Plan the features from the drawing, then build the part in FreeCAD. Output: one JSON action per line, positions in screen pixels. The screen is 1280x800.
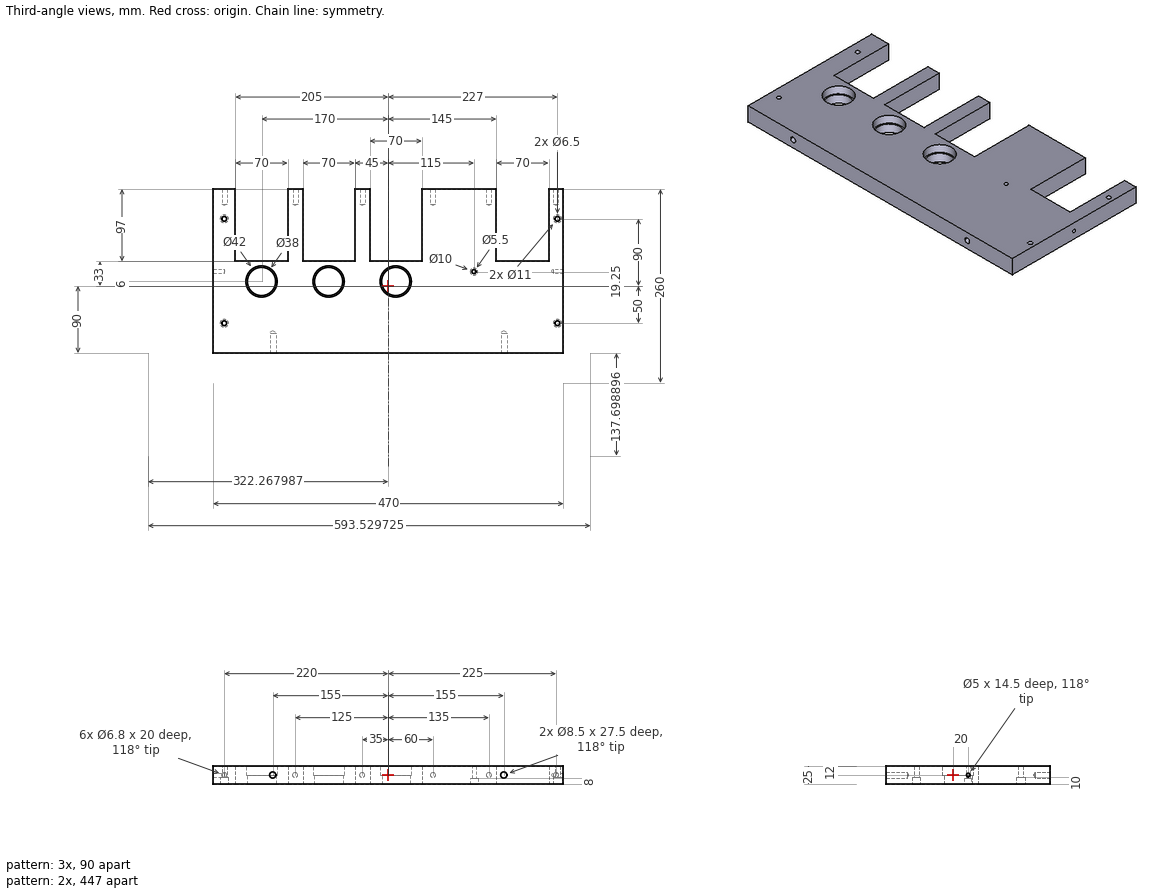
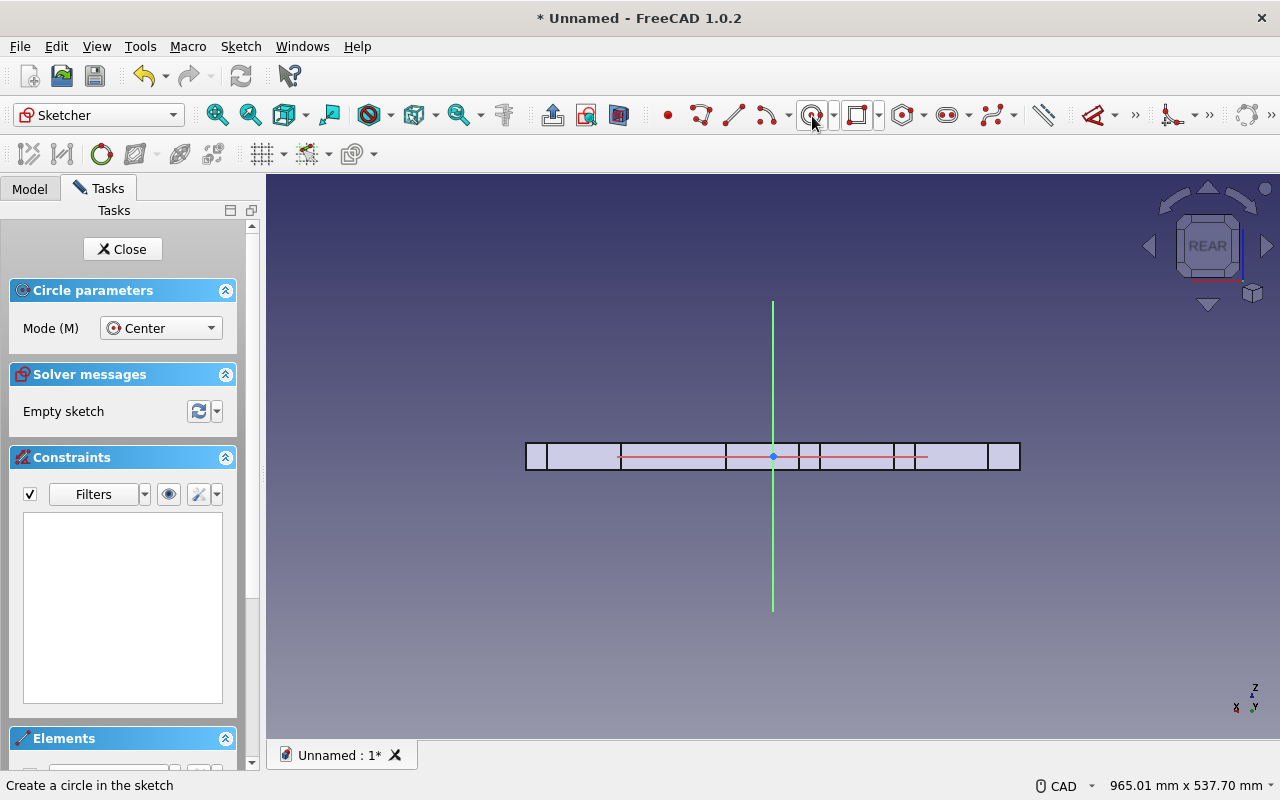
{"action": "scroll", "coordinate": [1004, 456], "scroll_direction": "up", "scroll_amount": 10}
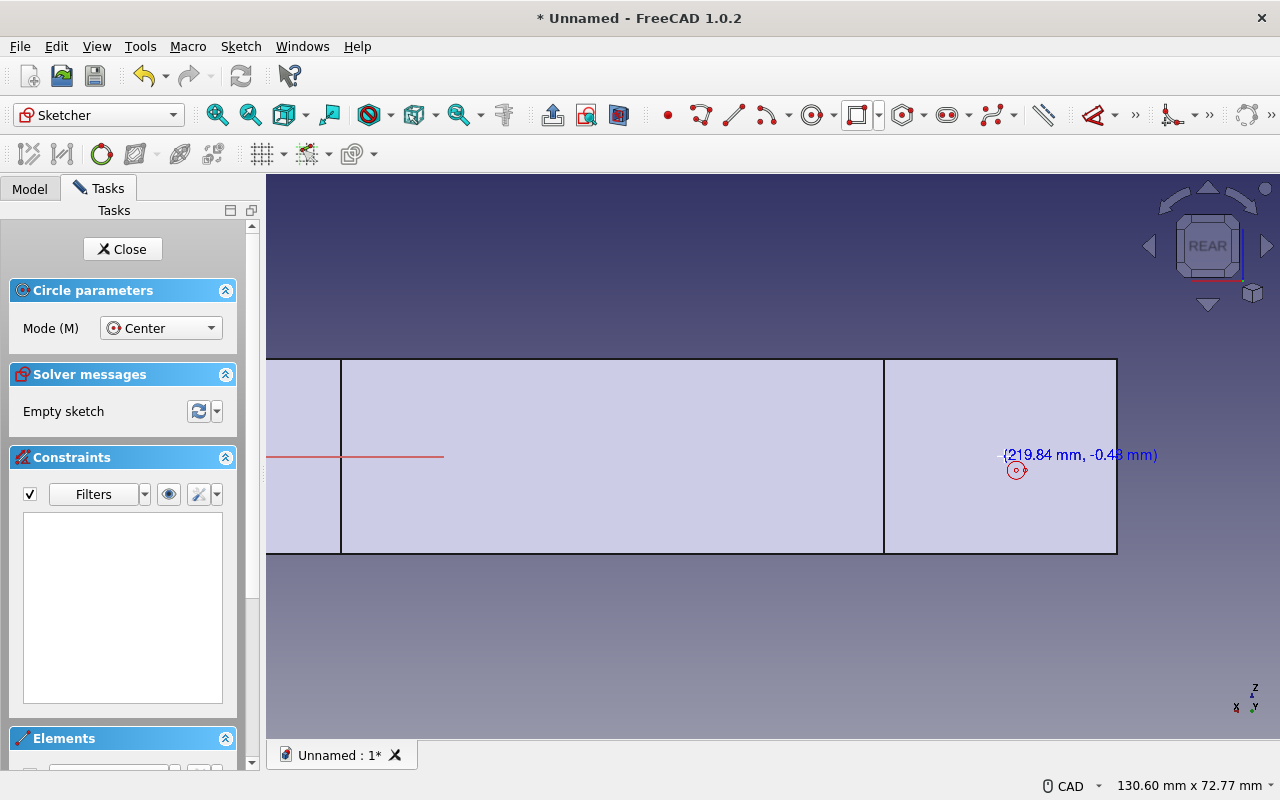
{"action": "scroll", "coordinate": [988, 457], "scroll_direction": "down", "scroll_amount": 9}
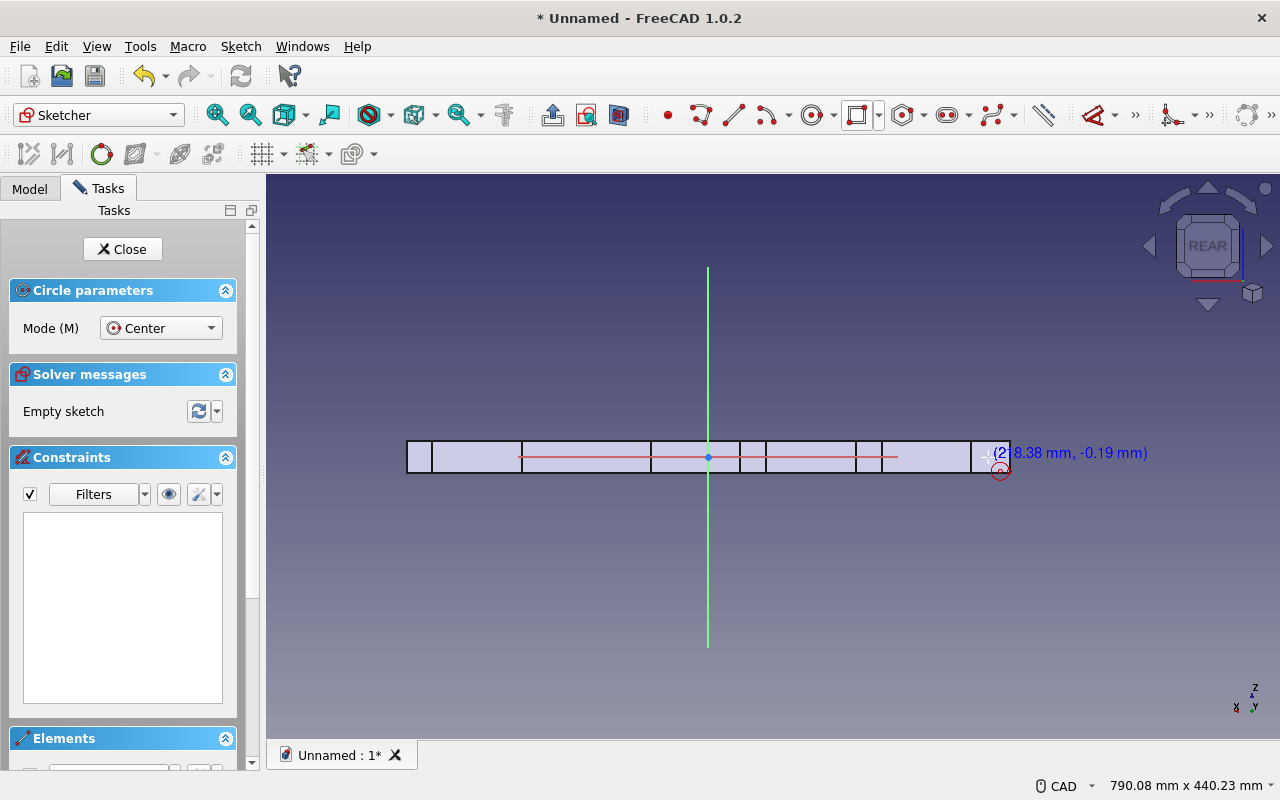
{"action": "left_click", "coordinate": [991, 457]}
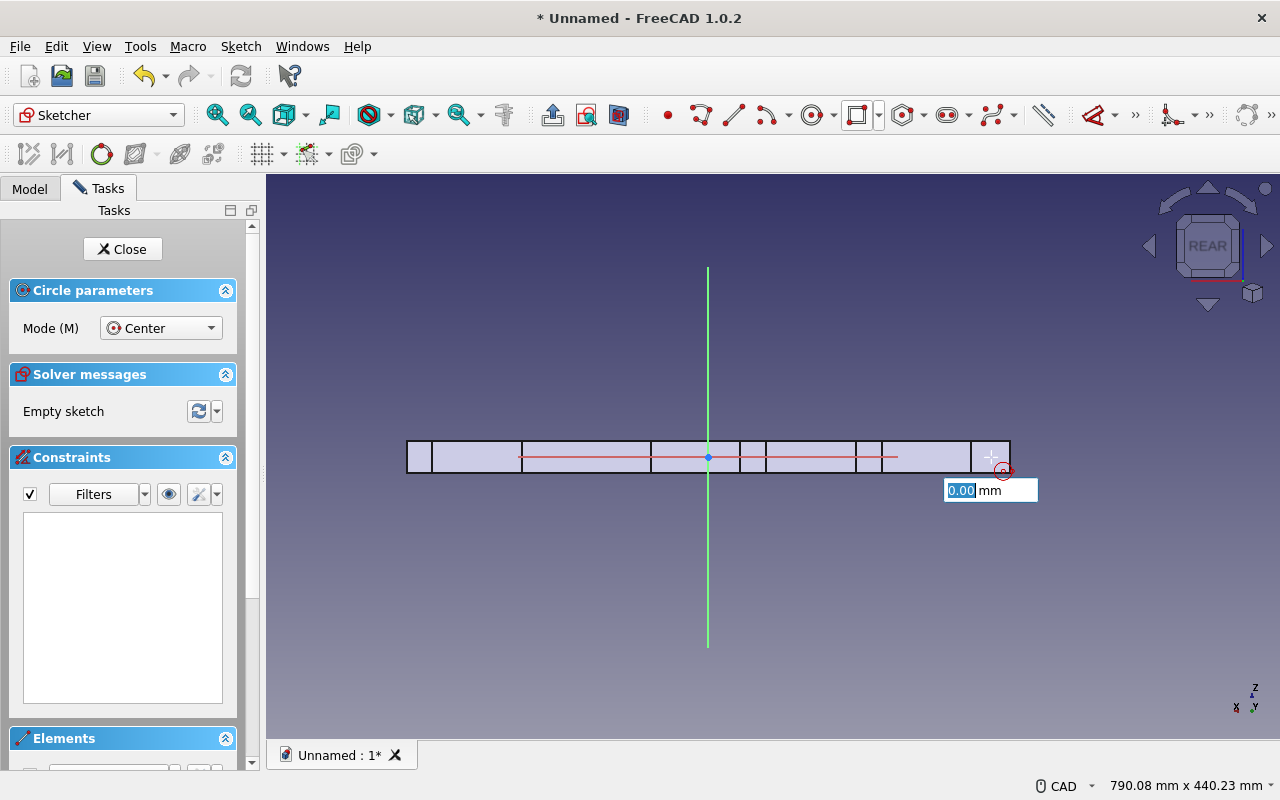
{"action": "scroll", "coordinate": [992, 453], "scroll_direction": "up", "scroll_amount": 7}
{"action": "mouse_move", "coordinate": [990, 452]}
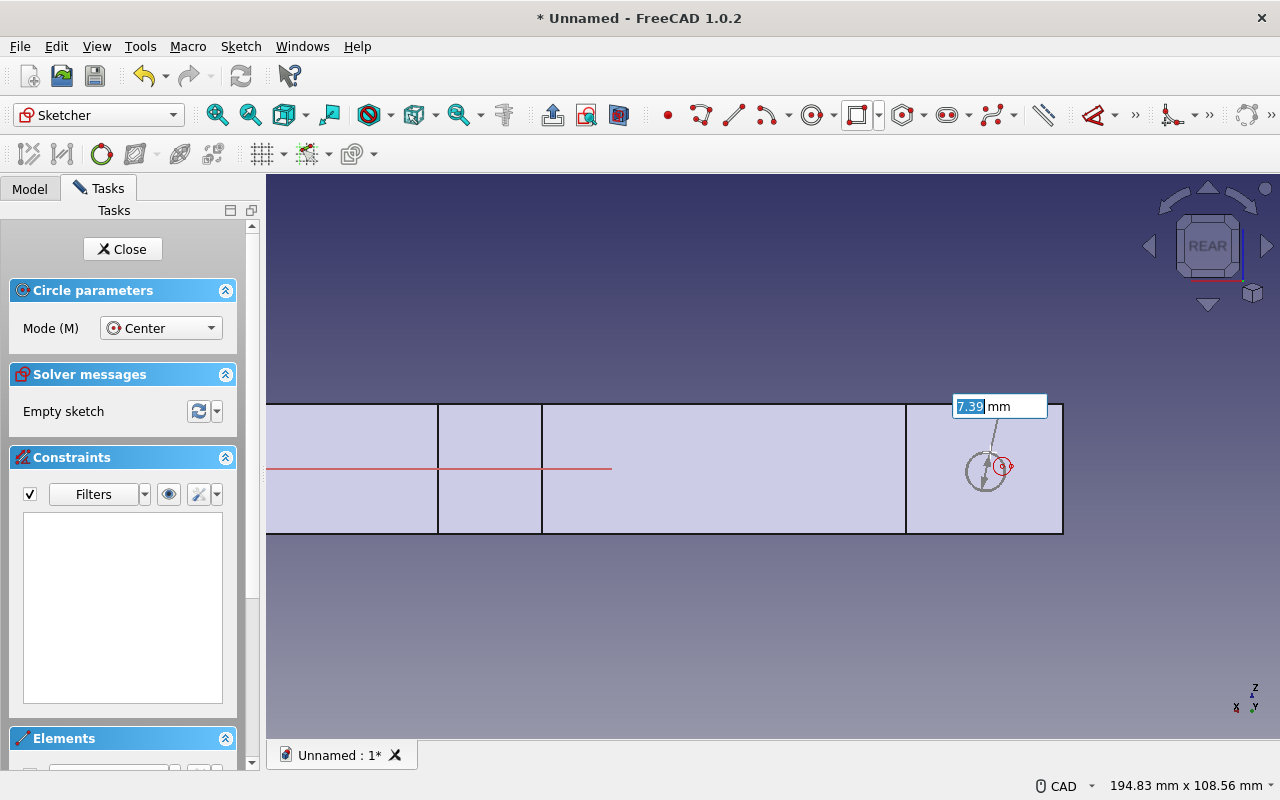
{"action": "type", "text": "6.8"}
{"action": "key", "text": "Return"}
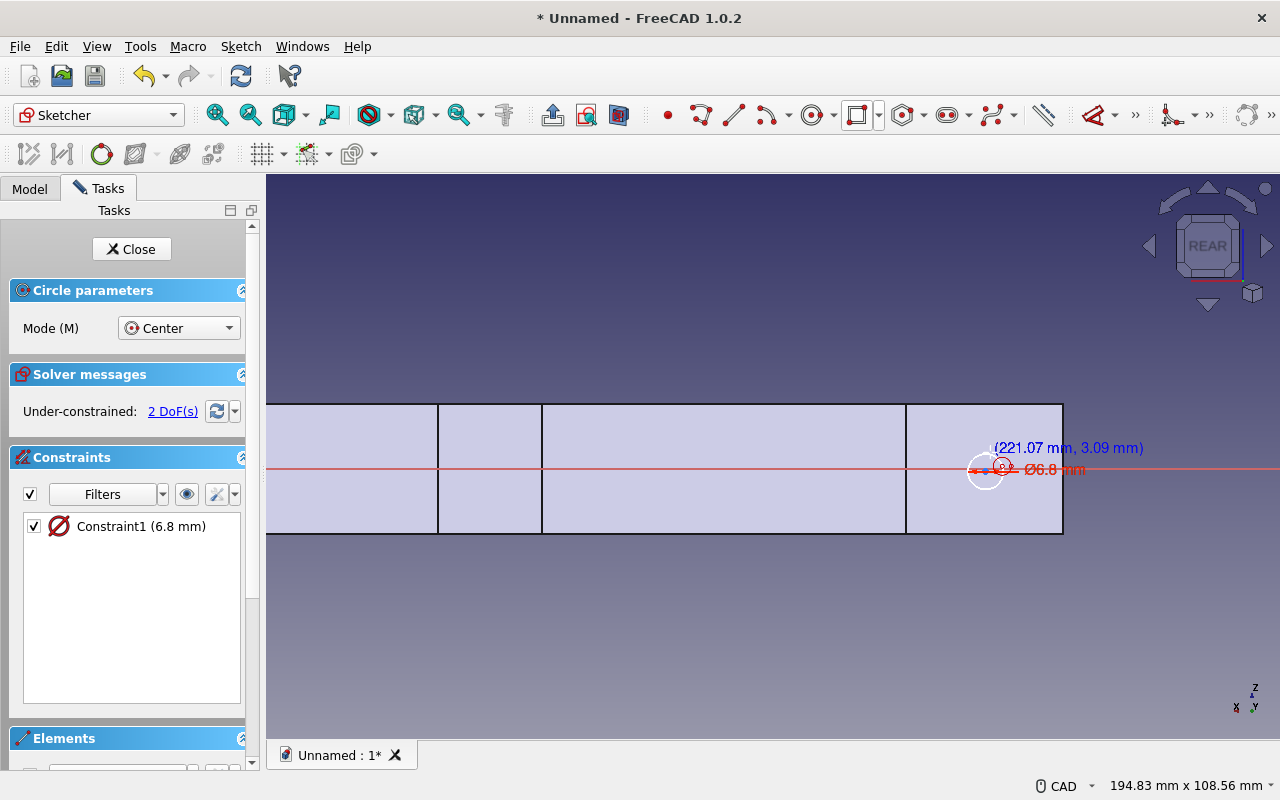
{"action": "scroll", "coordinate": [992, 452], "scroll_direction": "down", "scroll_amount": 7}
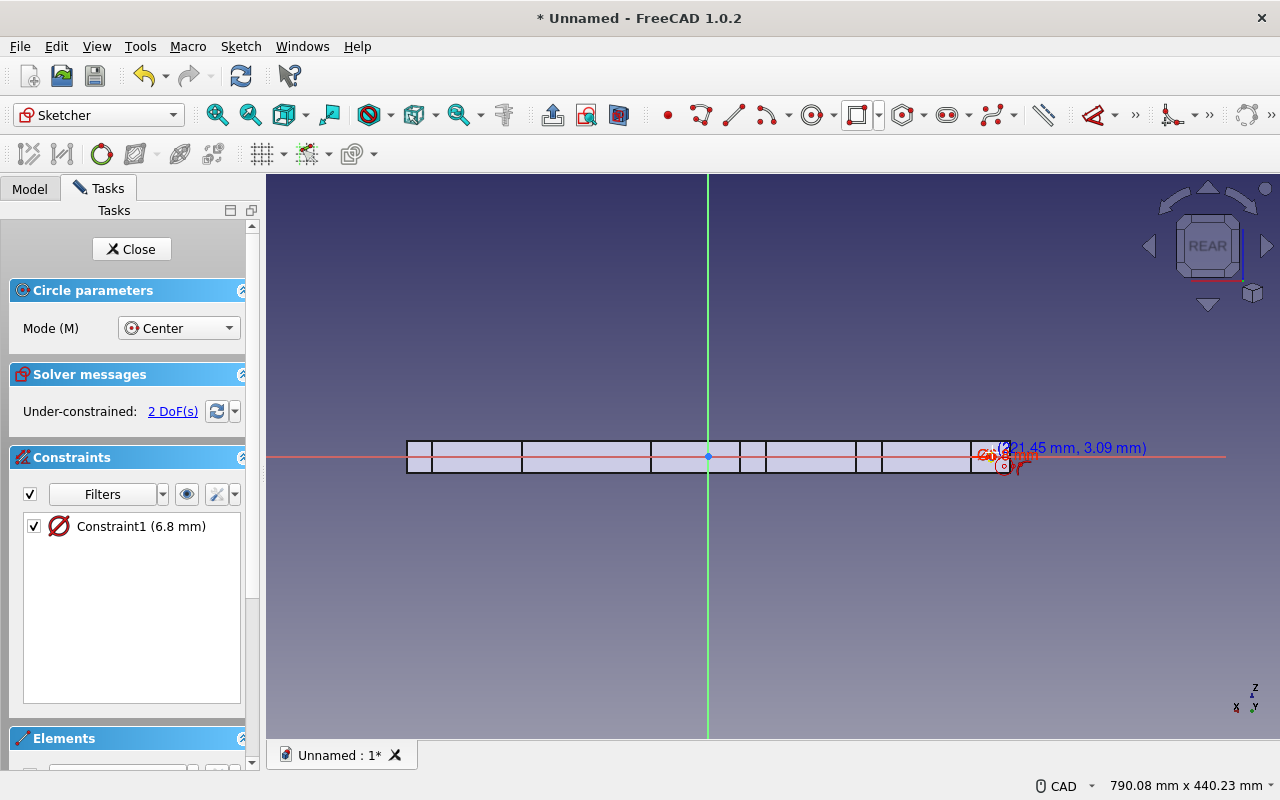
{"action": "scroll", "coordinate": [420, 457], "scroll_direction": "up", "scroll_amount": 9}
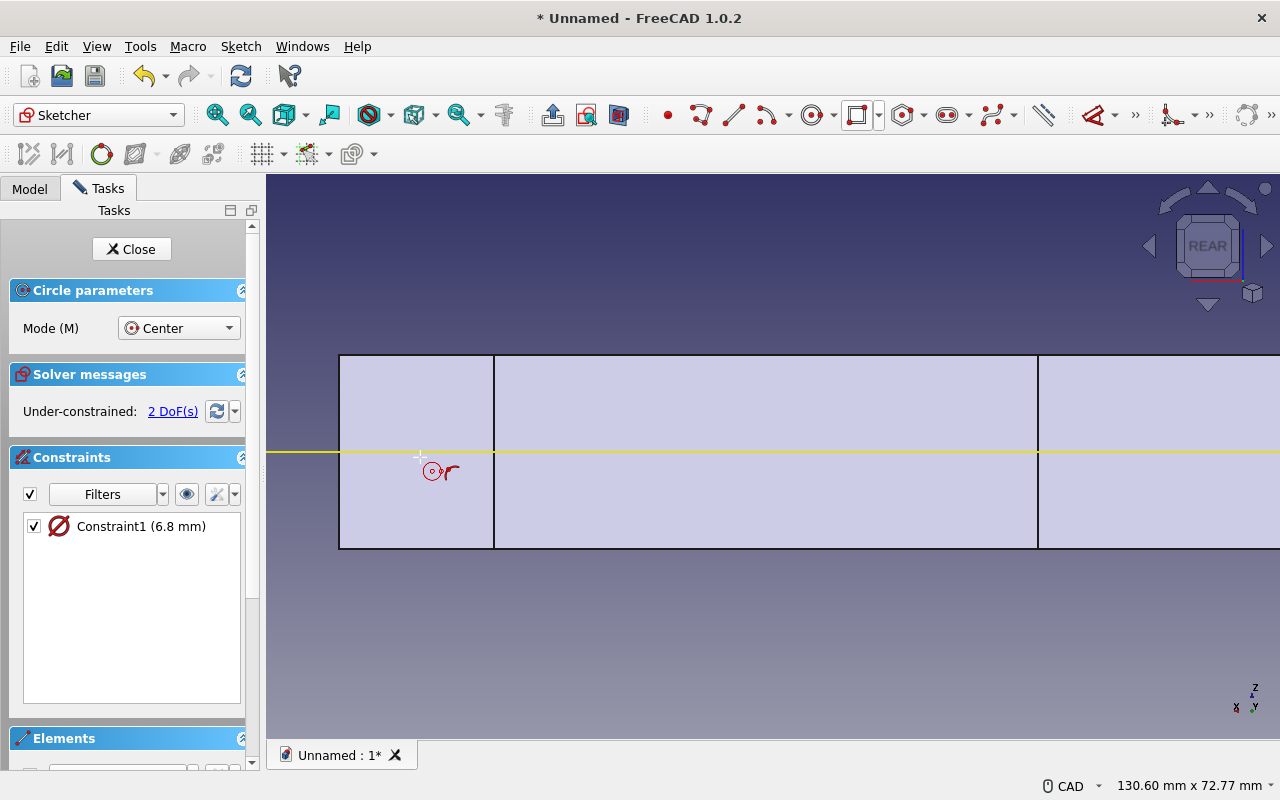
{"action": "scroll", "coordinate": [419, 457], "scroll_direction": "down", "scroll_amount": 9}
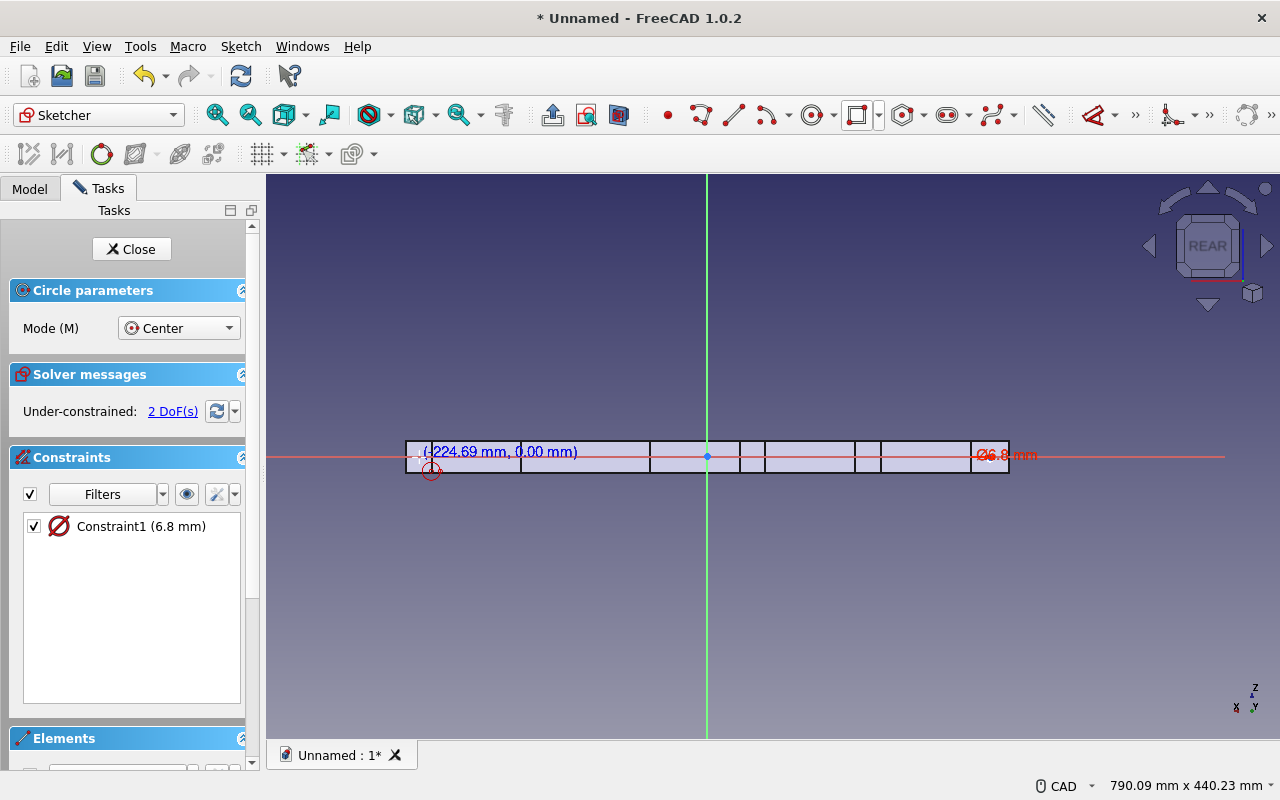
{"action": "left_click", "coordinate": [419, 457]}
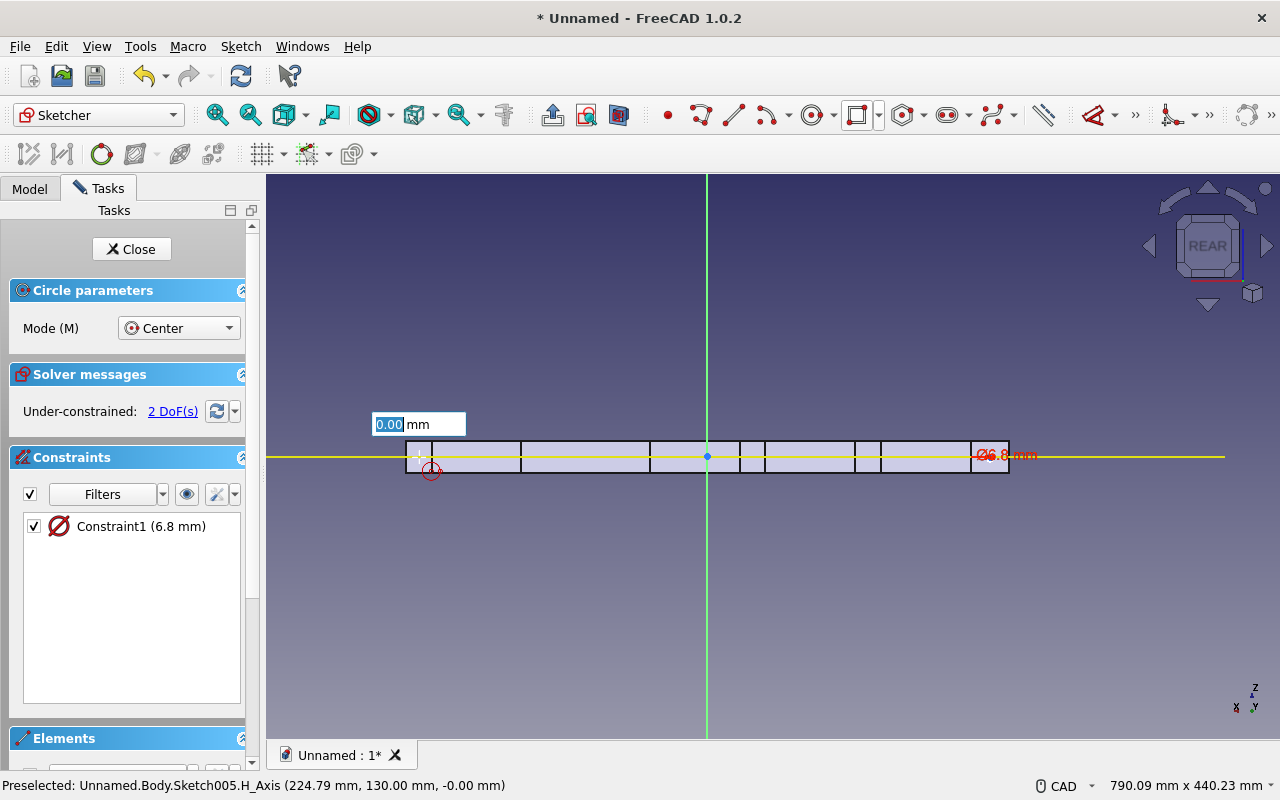
{"action": "scroll", "coordinate": [420, 452], "scroll_direction": "up", "scroll_amount": 7}
{"action": "mouse_move", "coordinate": [420, 452]}